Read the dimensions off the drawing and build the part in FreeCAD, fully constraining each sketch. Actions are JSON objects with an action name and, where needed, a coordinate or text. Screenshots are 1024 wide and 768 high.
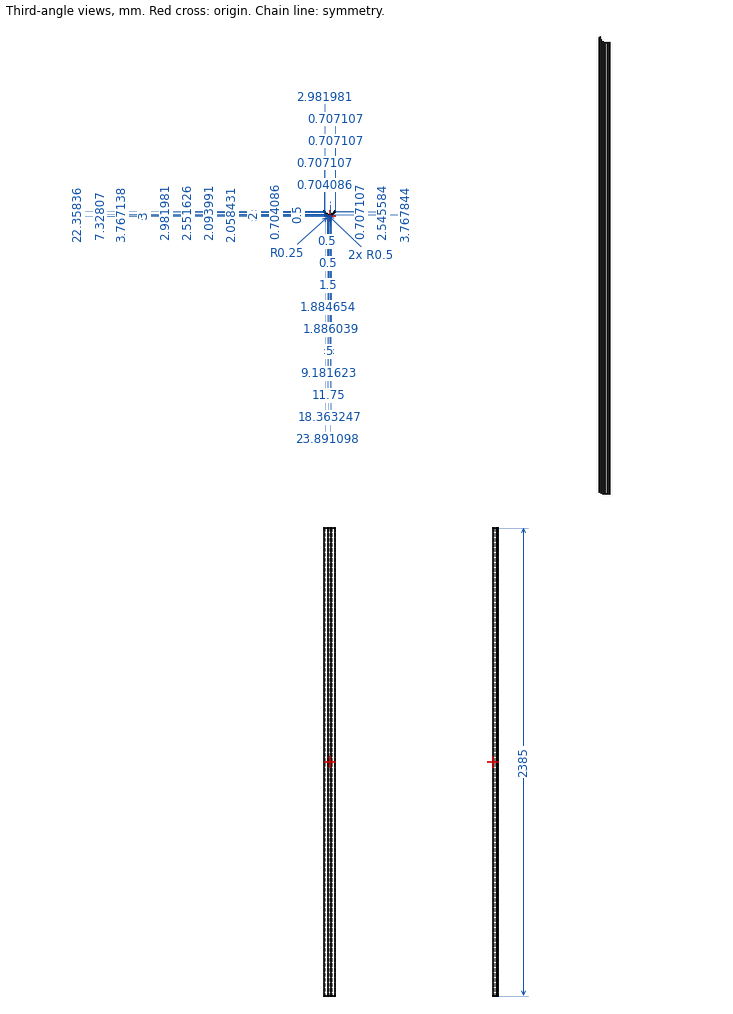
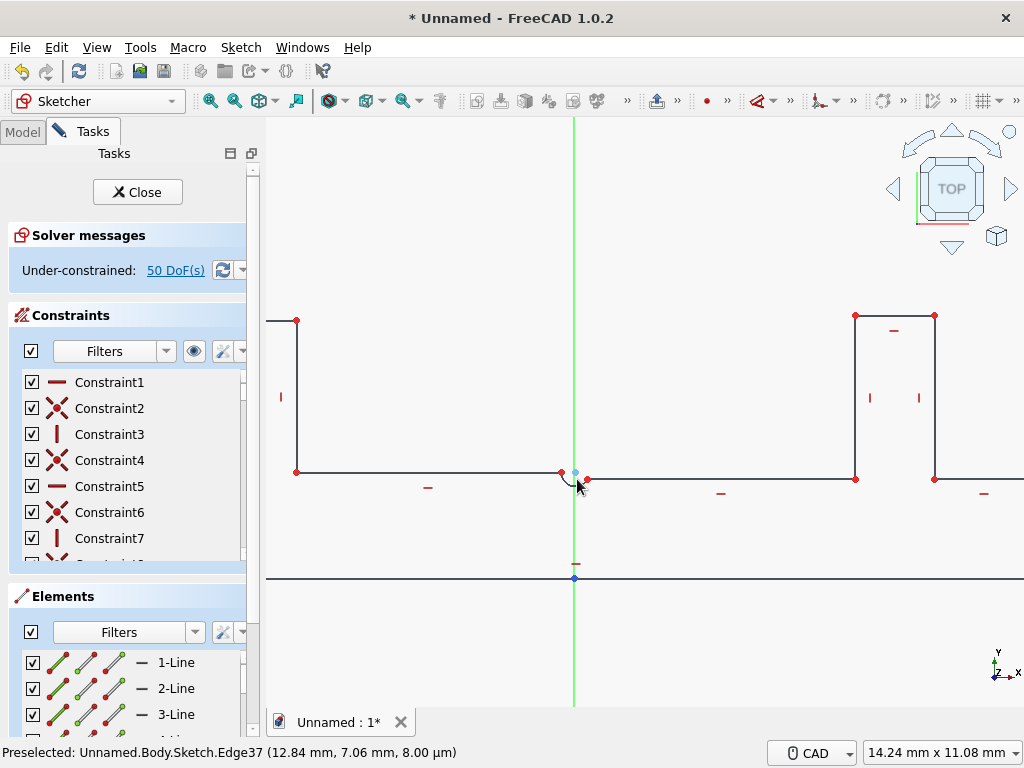
{"action": "left_click", "coordinate": [575, 472]}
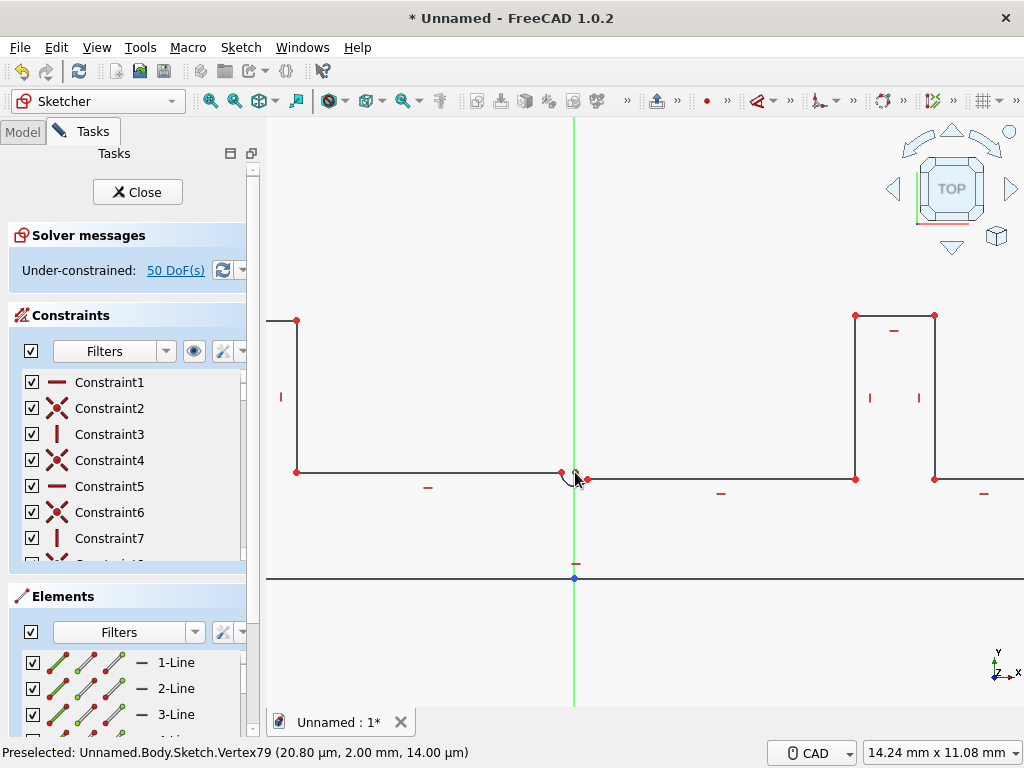
{"action": "left_click", "coordinate": [574, 641]}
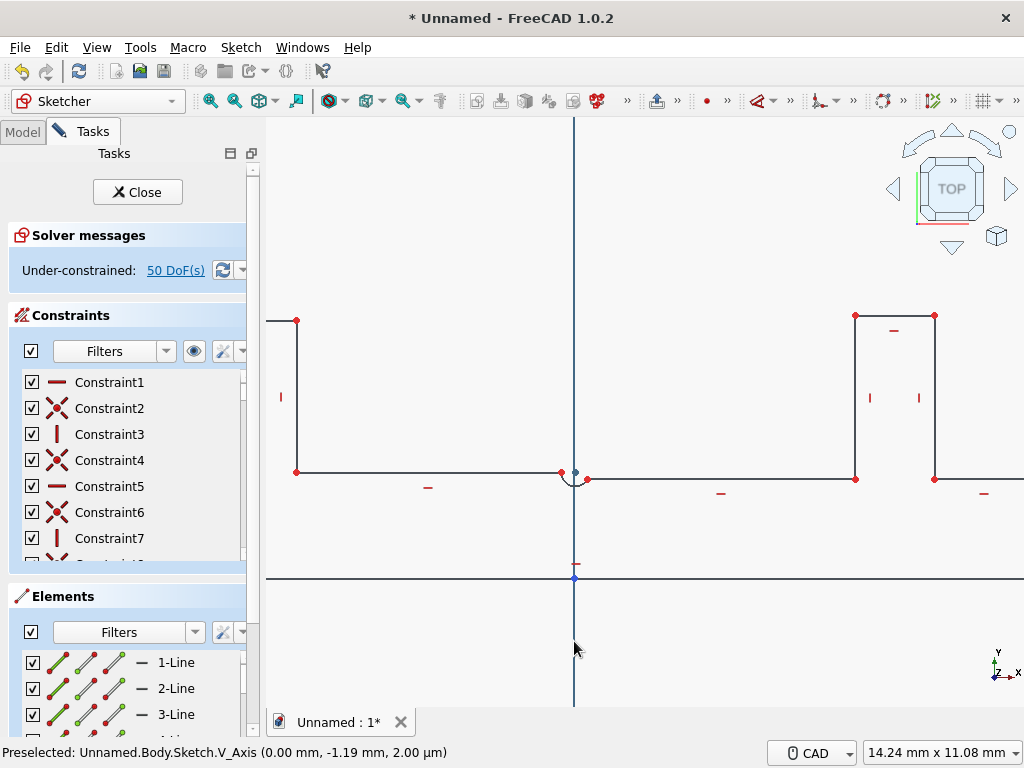
{"action": "key", "text": "c"}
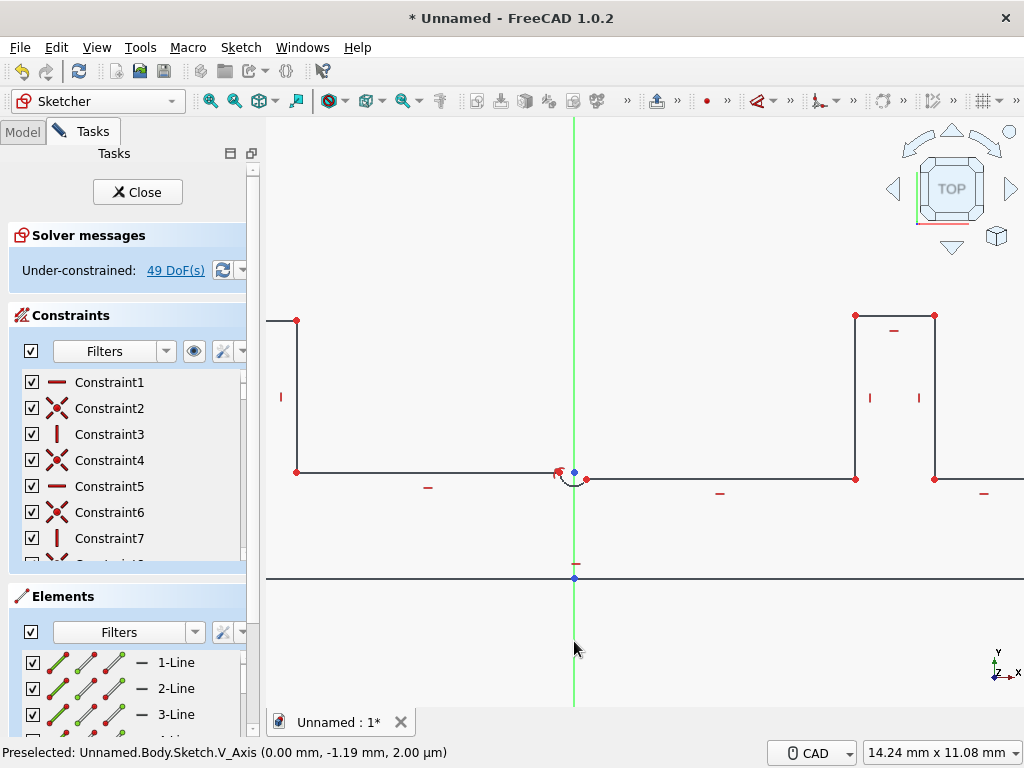
{"action": "scroll", "coordinate": [577, 479], "scroll_direction": "down", "scroll_amount": 10}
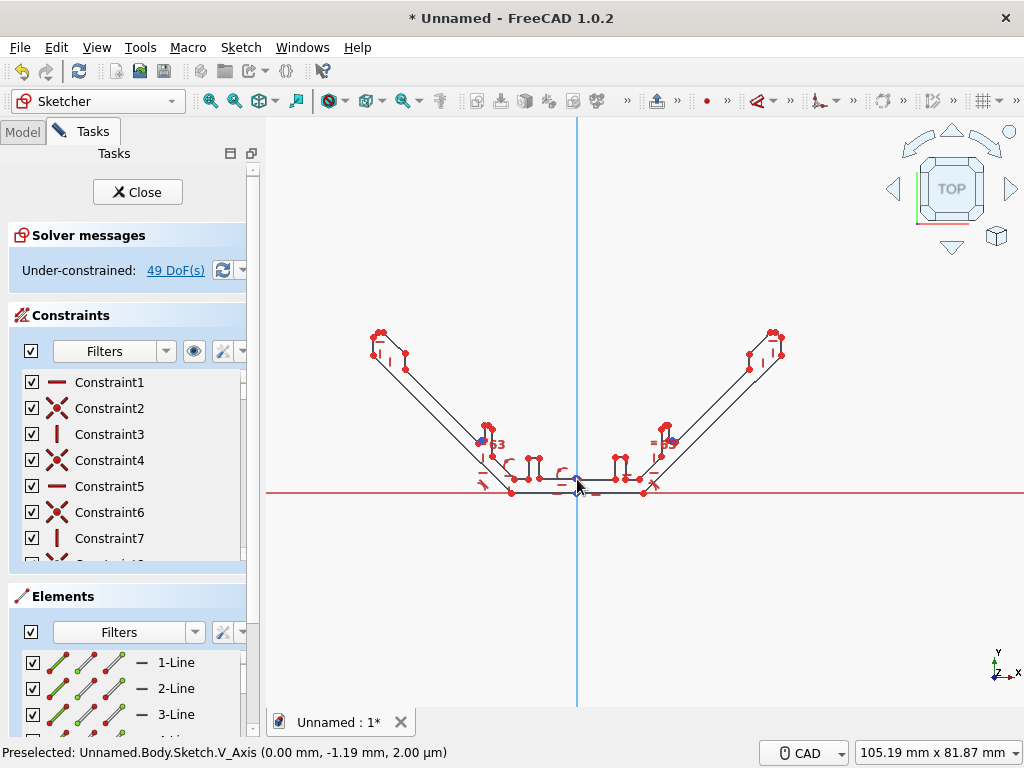
{"action": "scroll", "coordinate": [481, 440], "scroll_direction": "up", "scroll_amount": 7}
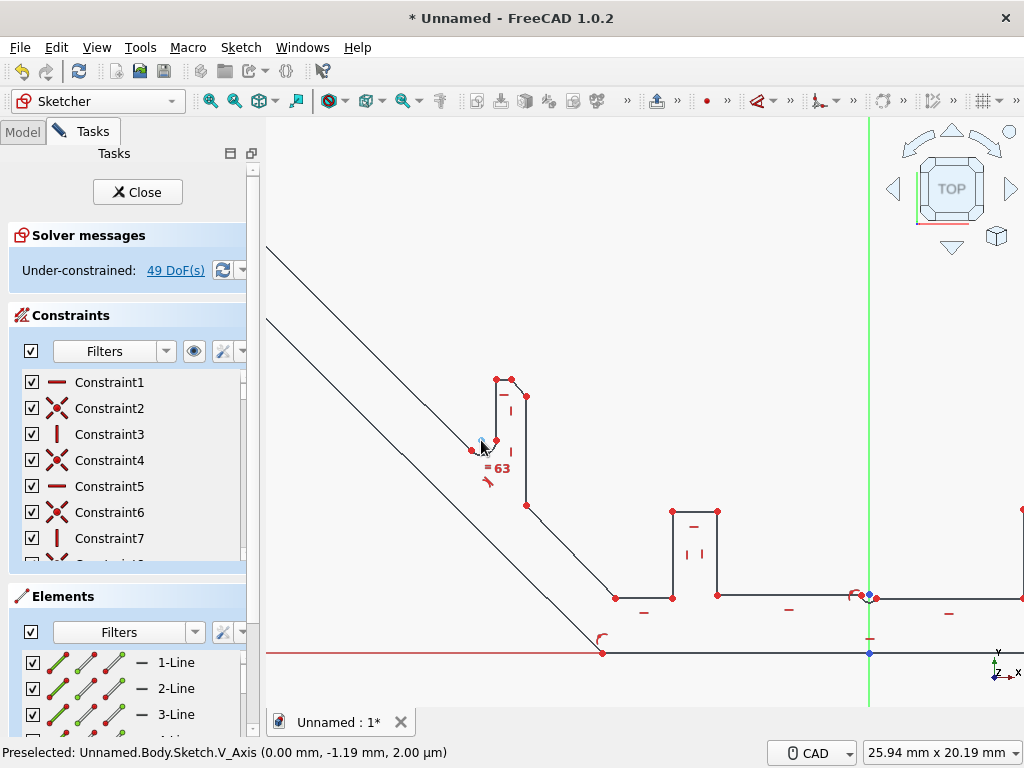
{"action": "left_click", "coordinate": [482, 440]}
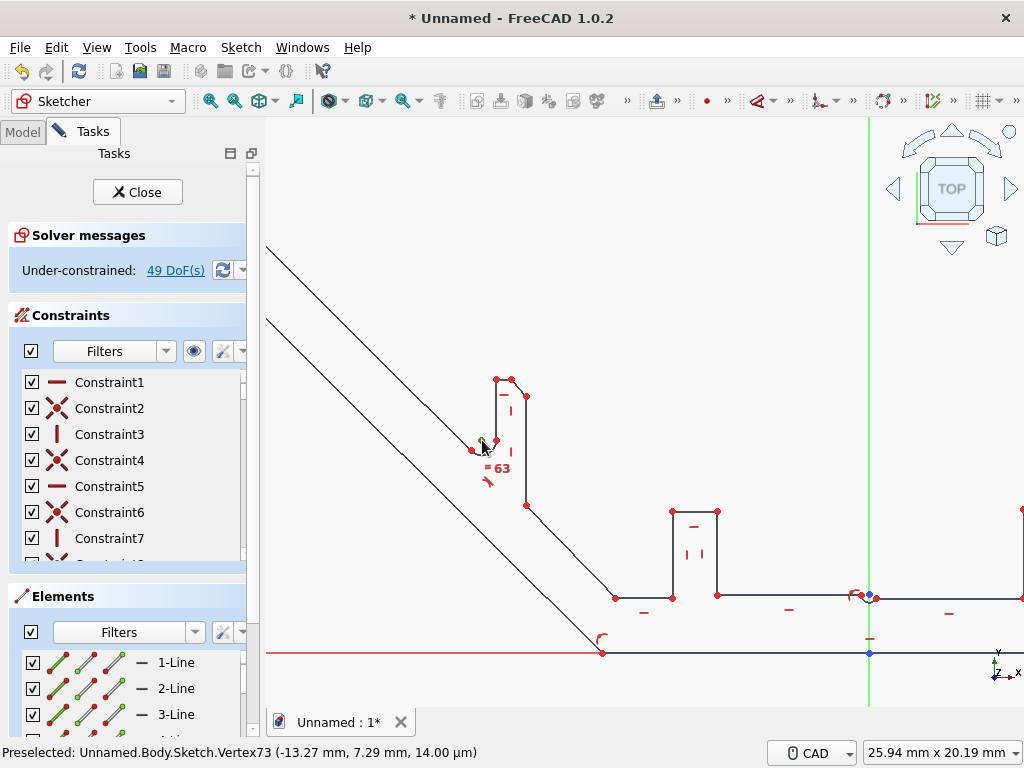
{"action": "scroll", "coordinate": [481, 440], "scroll_direction": "down", "scroll_amount": 7}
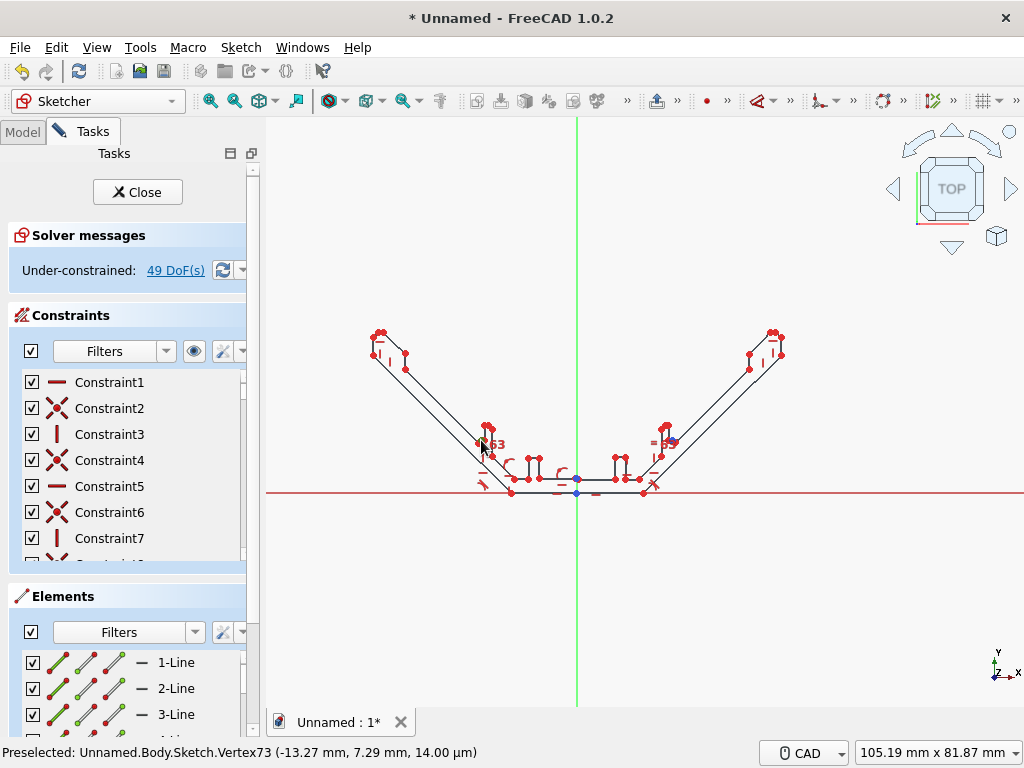
{"action": "scroll", "coordinate": [673, 440], "scroll_direction": "up", "scroll_amount": 7}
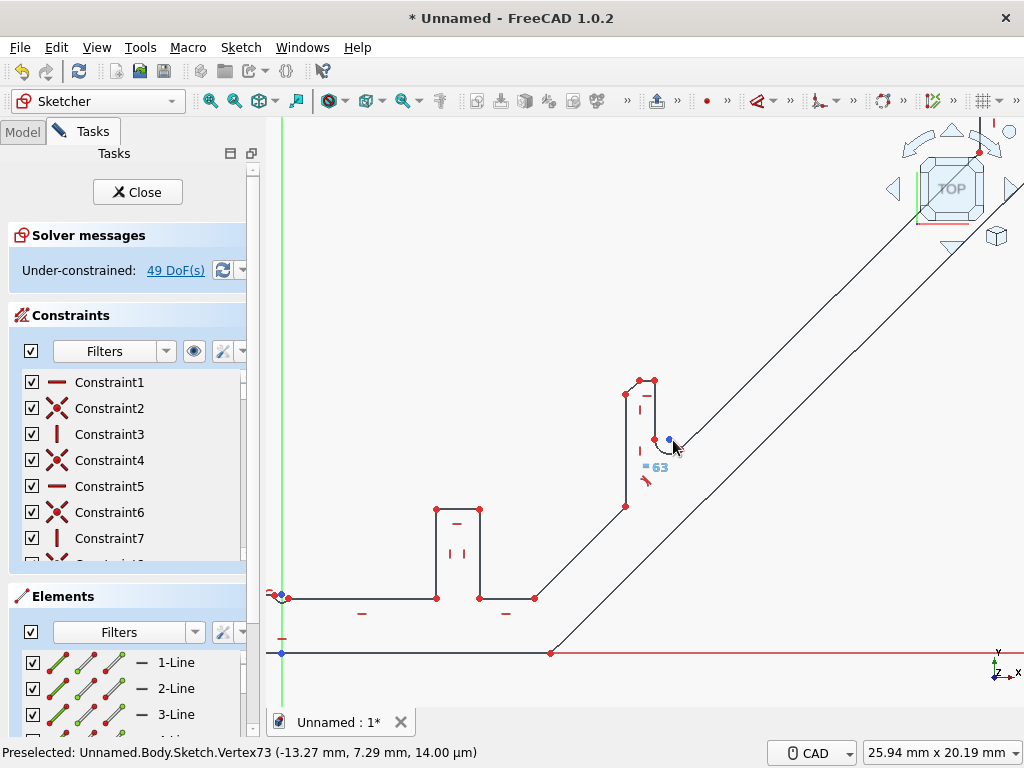
{"action": "left_click", "coordinate": [670, 439]}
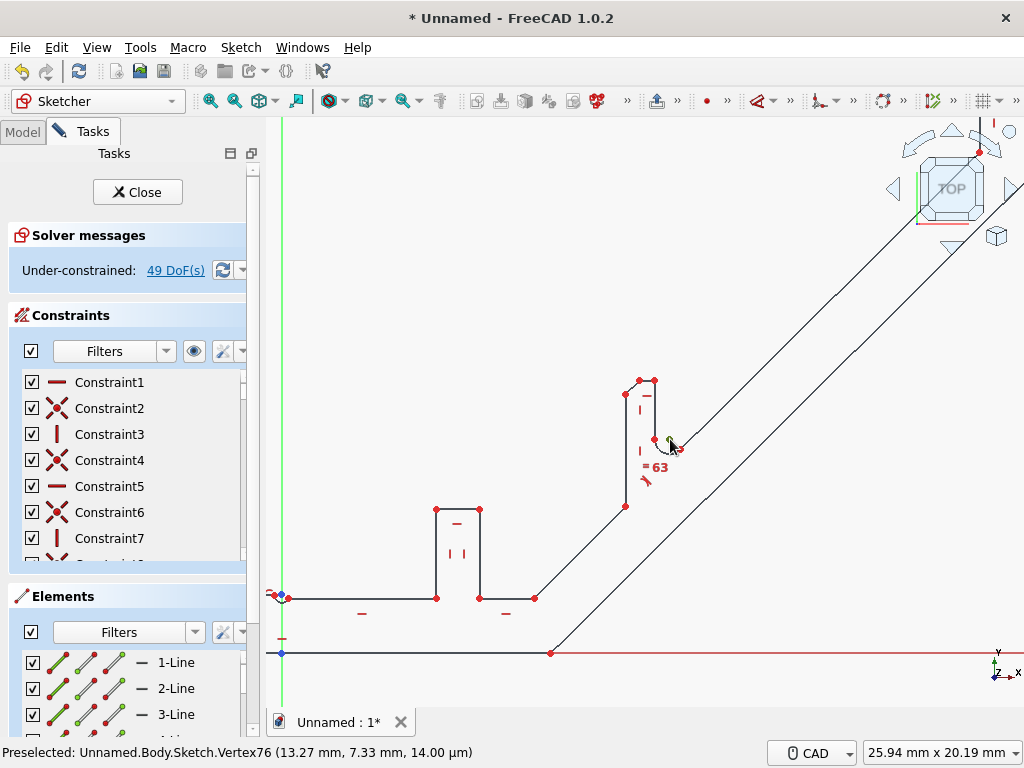
{"action": "scroll", "coordinate": [673, 440], "scroll_direction": "down", "scroll_amount": 7}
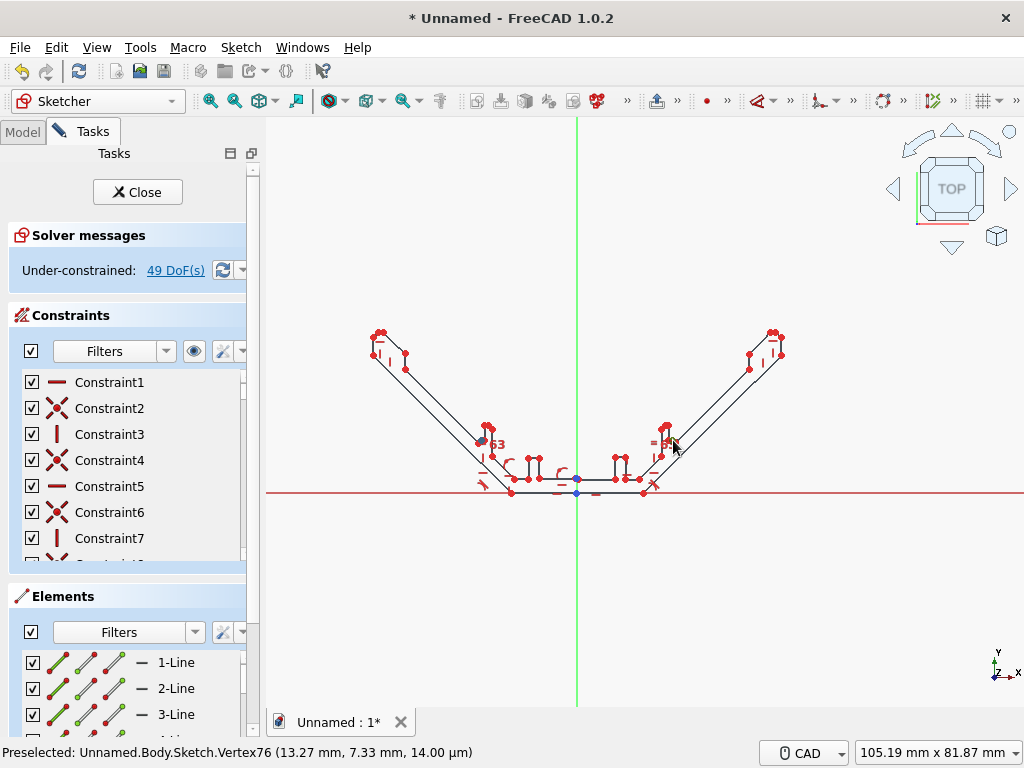
{"action": "left_click", "coordinate": [577, 641]}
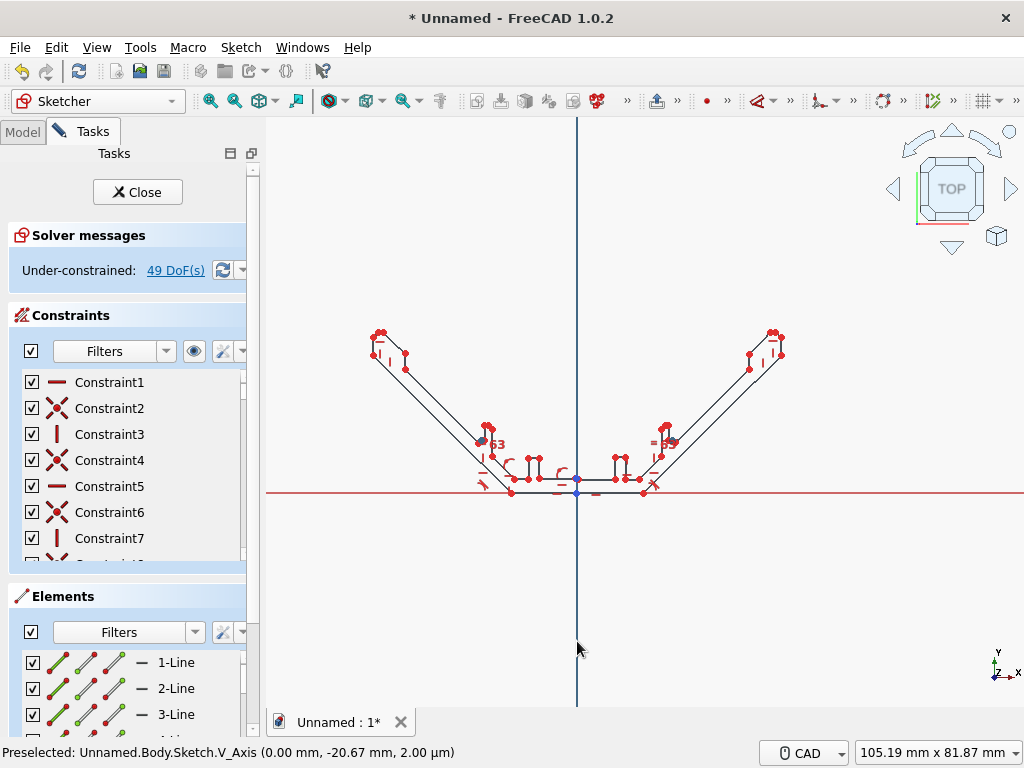
{"action": "key", "text": "s"}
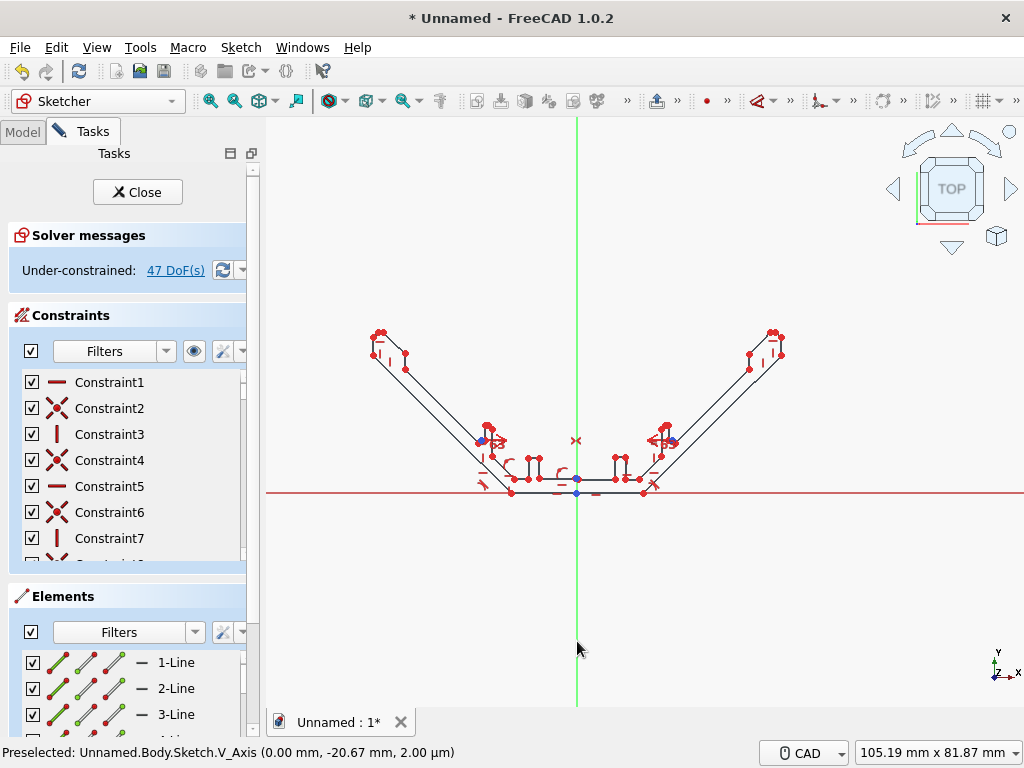
{"action": "scroll", "coordinate": [378, 333], "scroll_direction": "up", "scroll_amount": 5}